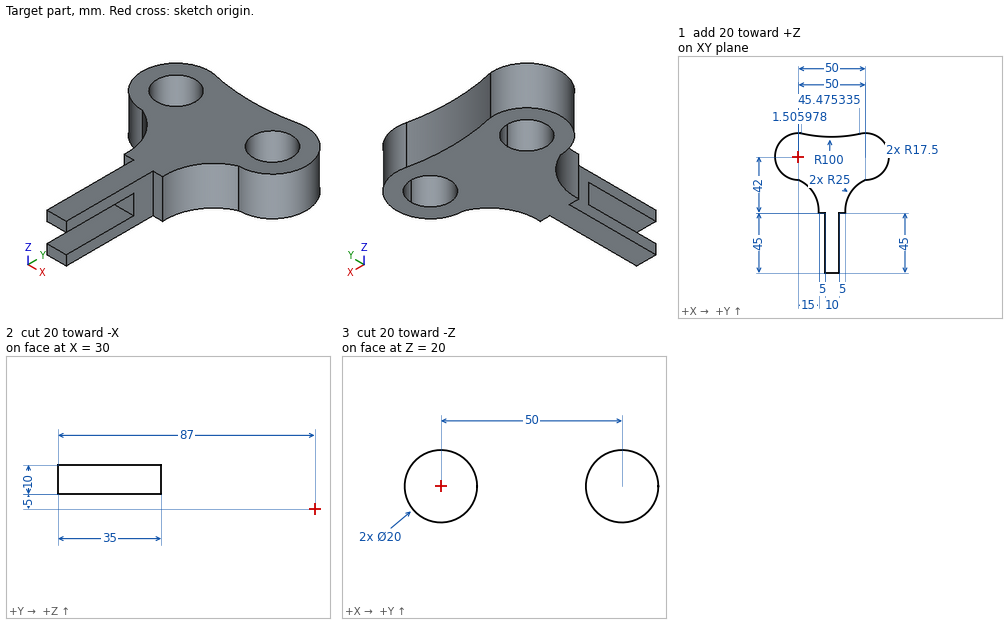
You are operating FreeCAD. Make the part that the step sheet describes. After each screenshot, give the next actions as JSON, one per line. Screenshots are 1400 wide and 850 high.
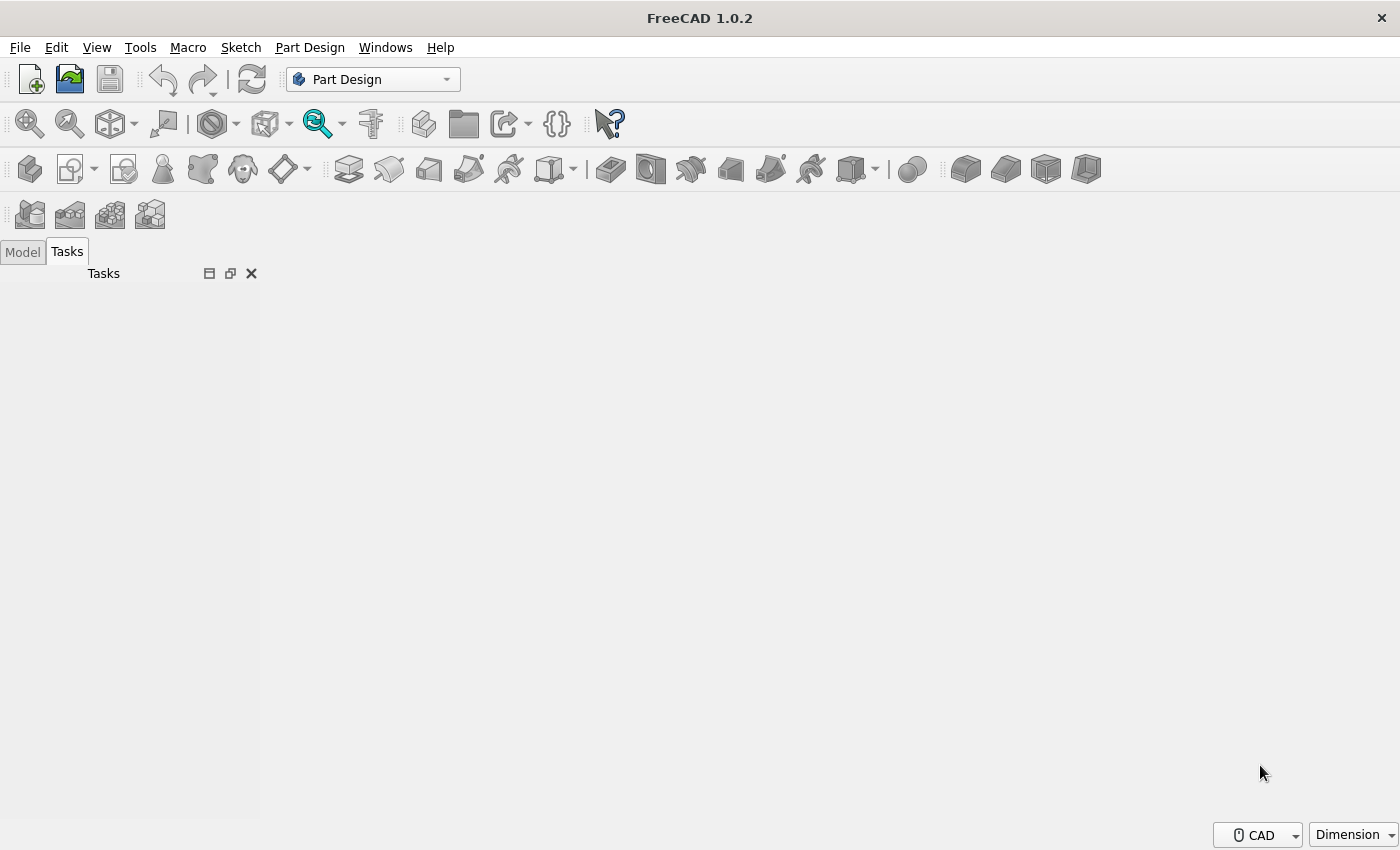
{"action": "left_click", "coordinate": [30, 80]}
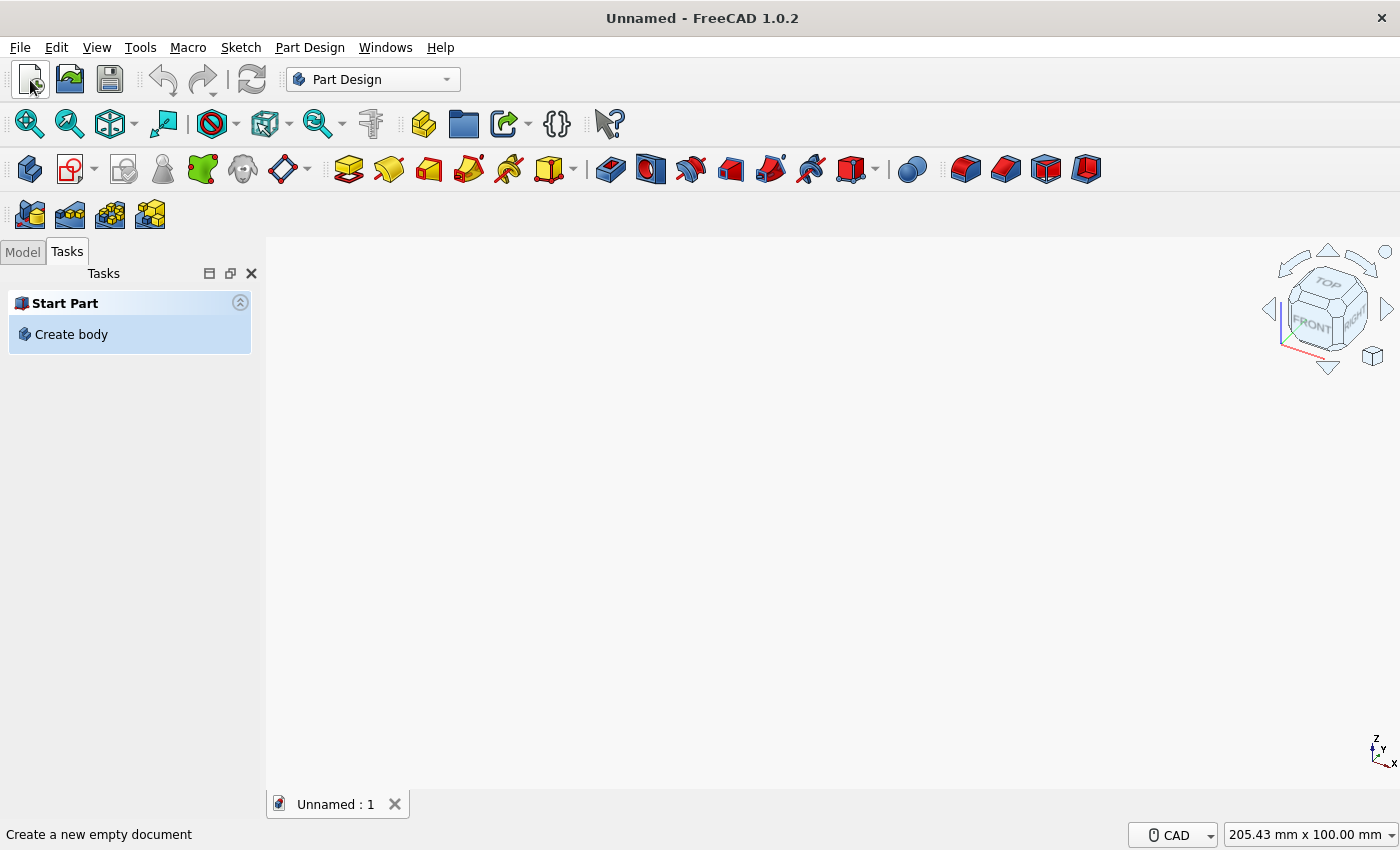
{"action": "left_click", "coordinate": [70, 170]}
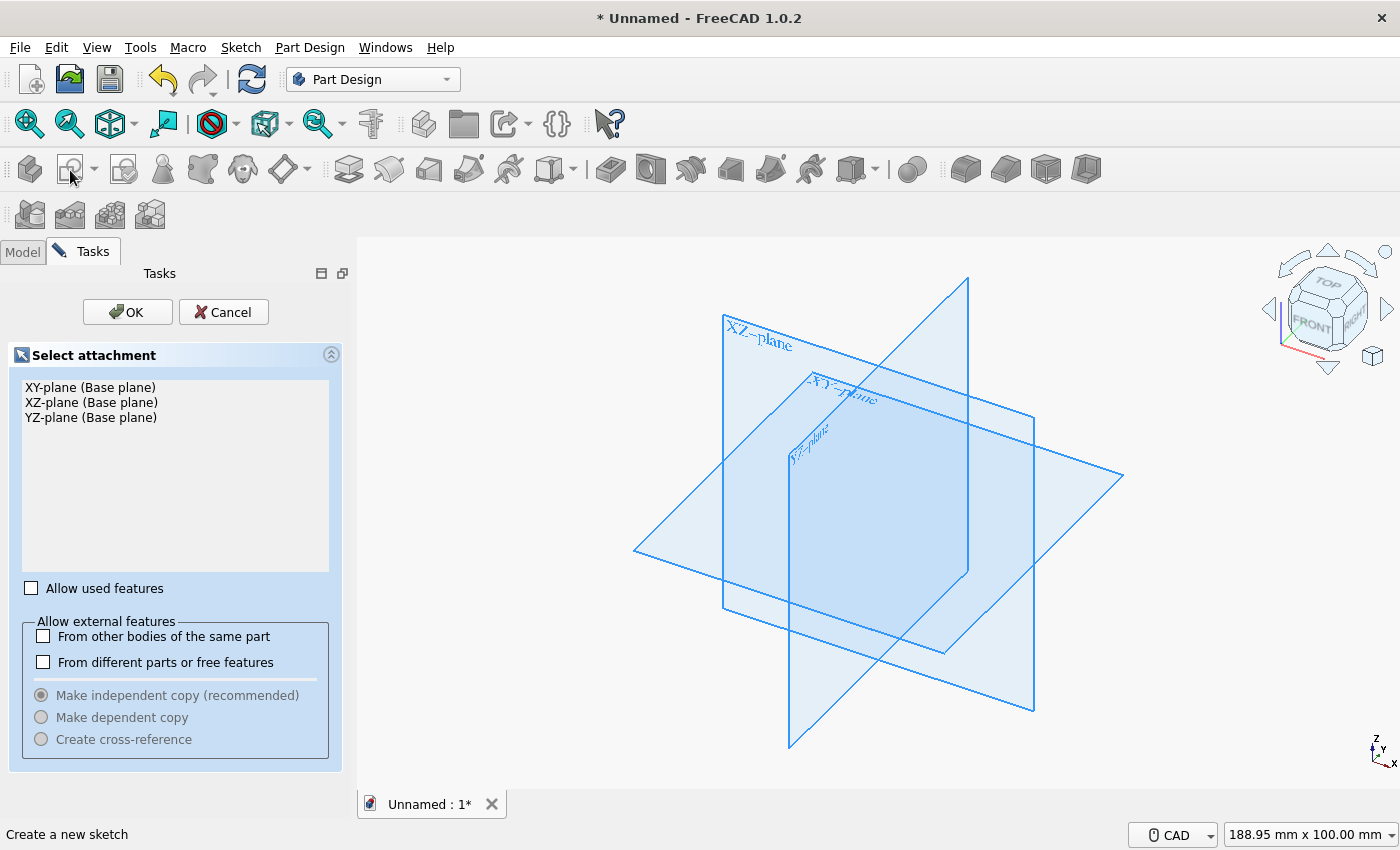
{"action": "left_click", "coordinate": [82, 388]}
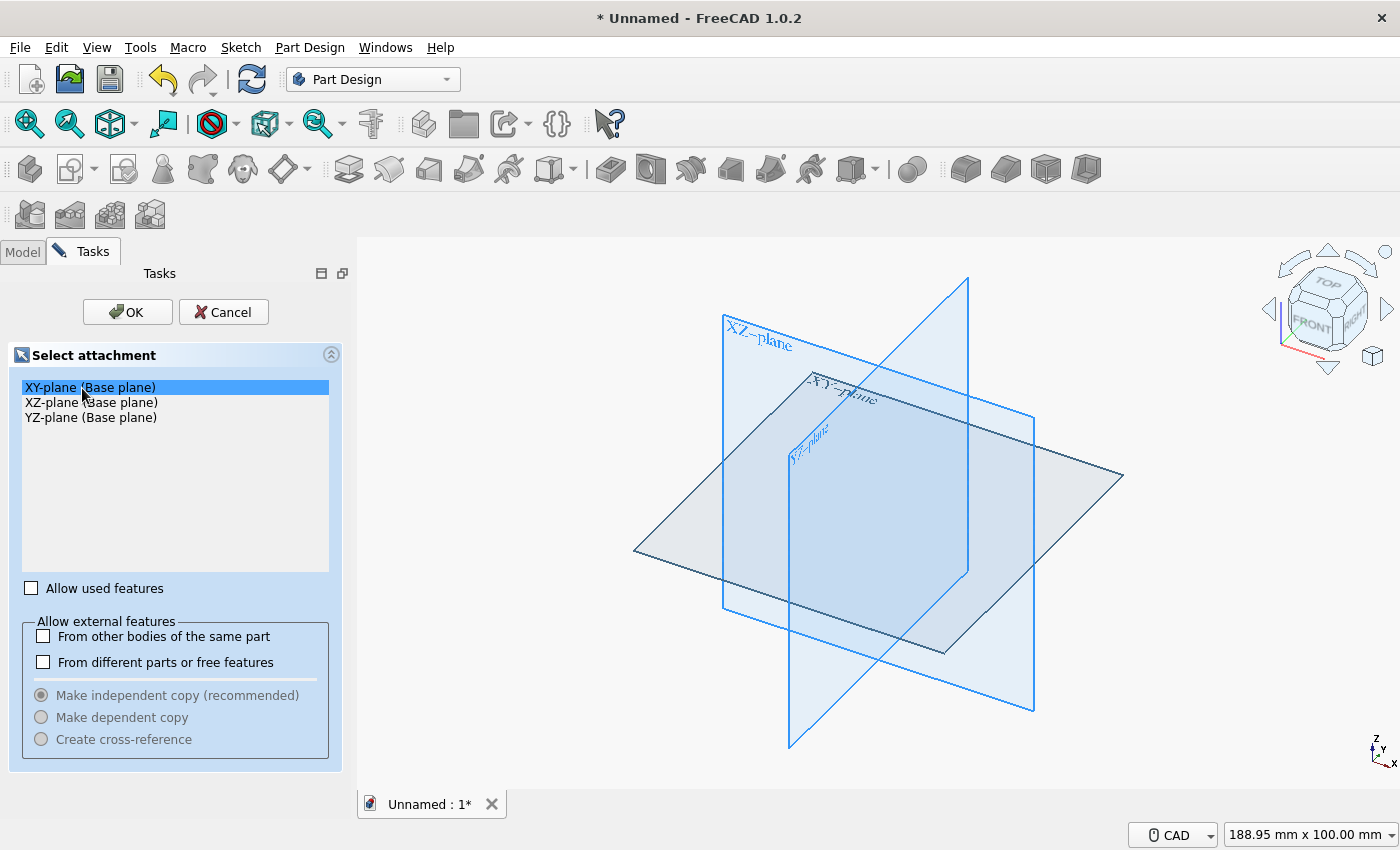
{"action": "left_click", "coordinate": [128, 312]}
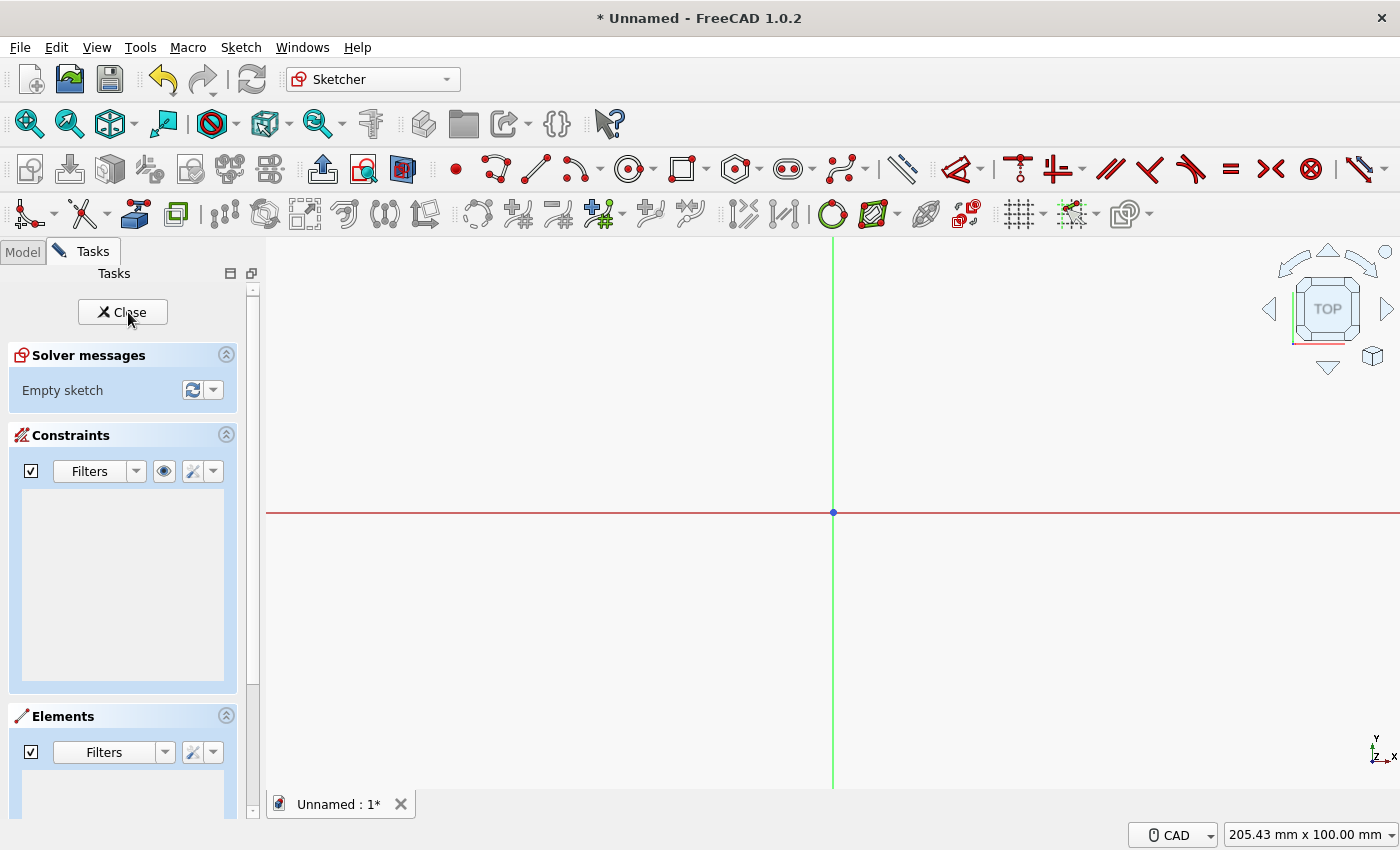
{"action": "scroll", "coordinate": [514, 279], "scroll_direction": "down", "scroll_amount": 3}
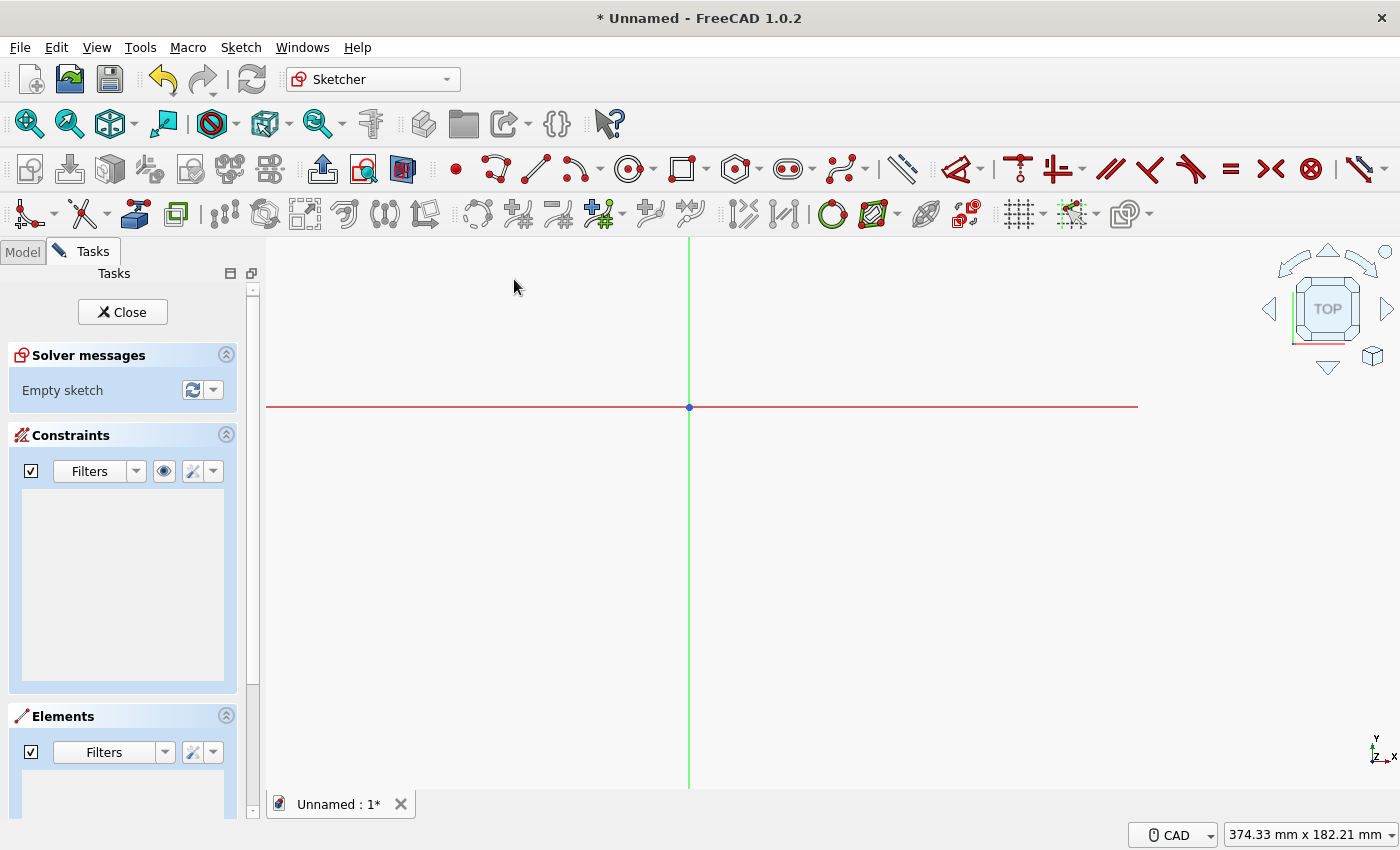
{"action": "left_click", "coordinate": [496, 170]}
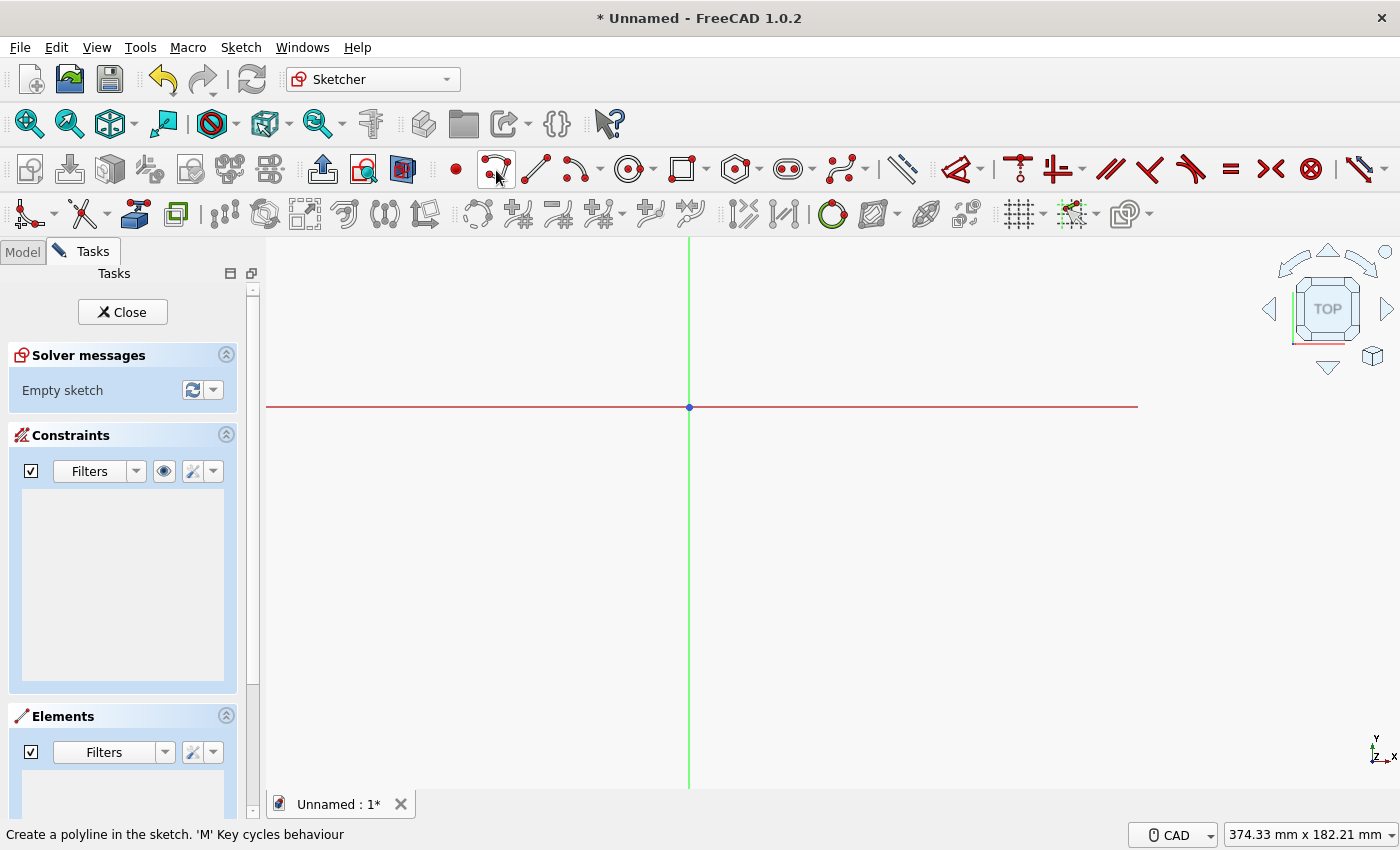
{"action": "left_click", "coordinate": [735, 535]}
{"action": "left_click", "coordinate": [750, 535]}
{"action": "left_click", "coordinate": [750, 671]}
{"action": "left_click", "coordinate": [780, 671]}
{"action": "left_click", "coordinate": [780, 535]}
{"action": "left_click", "coordinate": [795, 535]}
{"action": "right_click", "coordinate": [795, 535]}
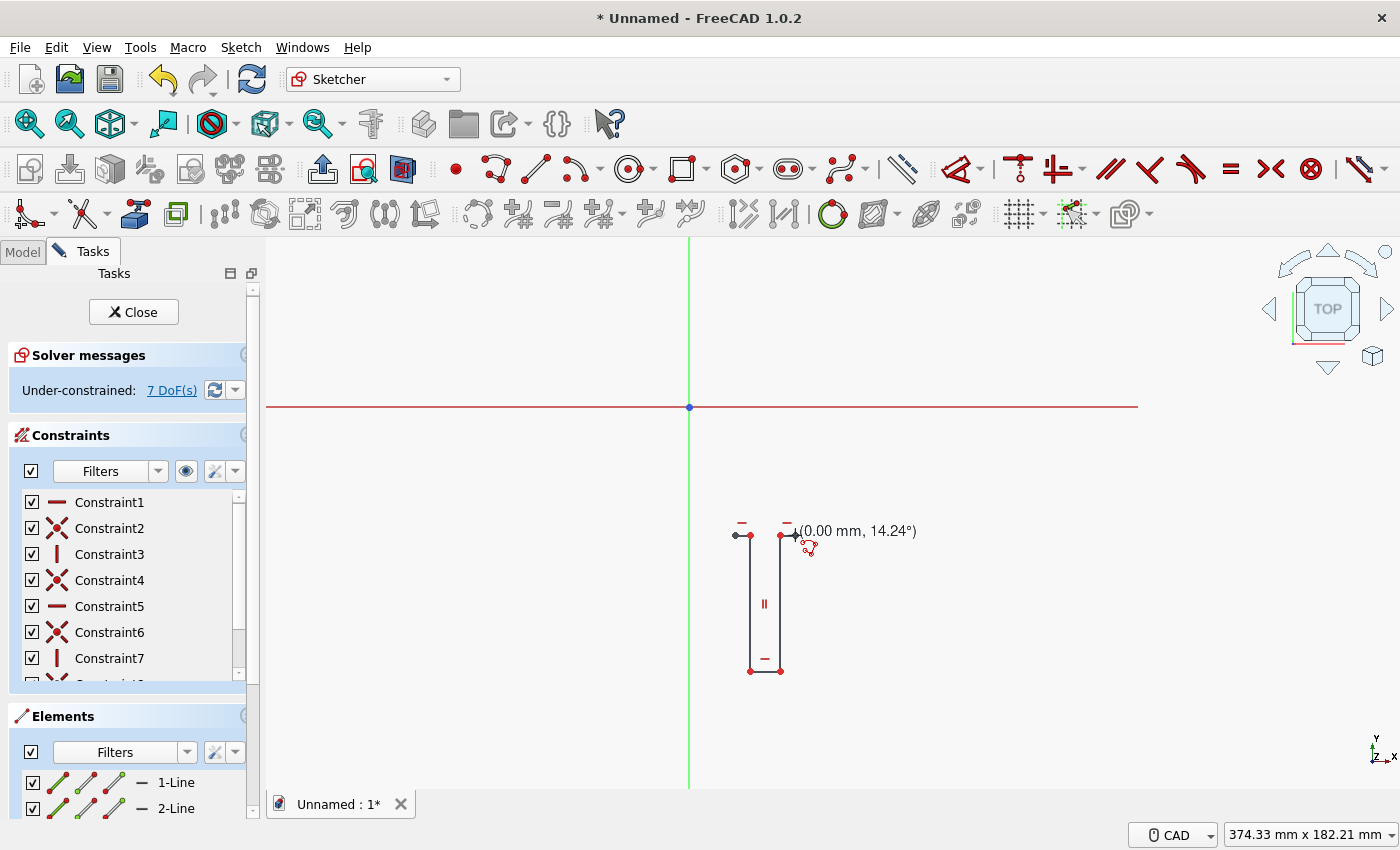
{"action": "key", "text": "g 3 a"}